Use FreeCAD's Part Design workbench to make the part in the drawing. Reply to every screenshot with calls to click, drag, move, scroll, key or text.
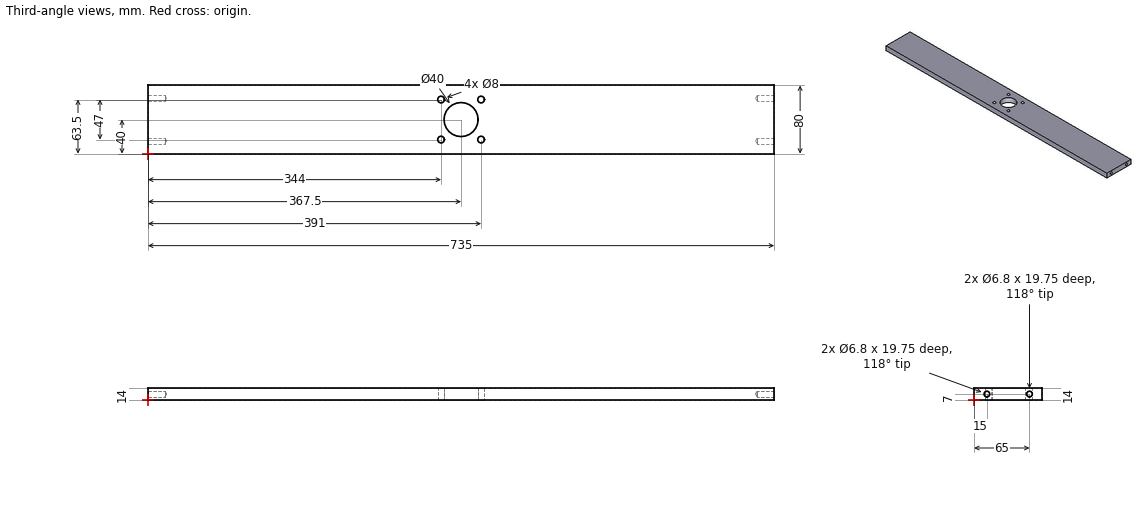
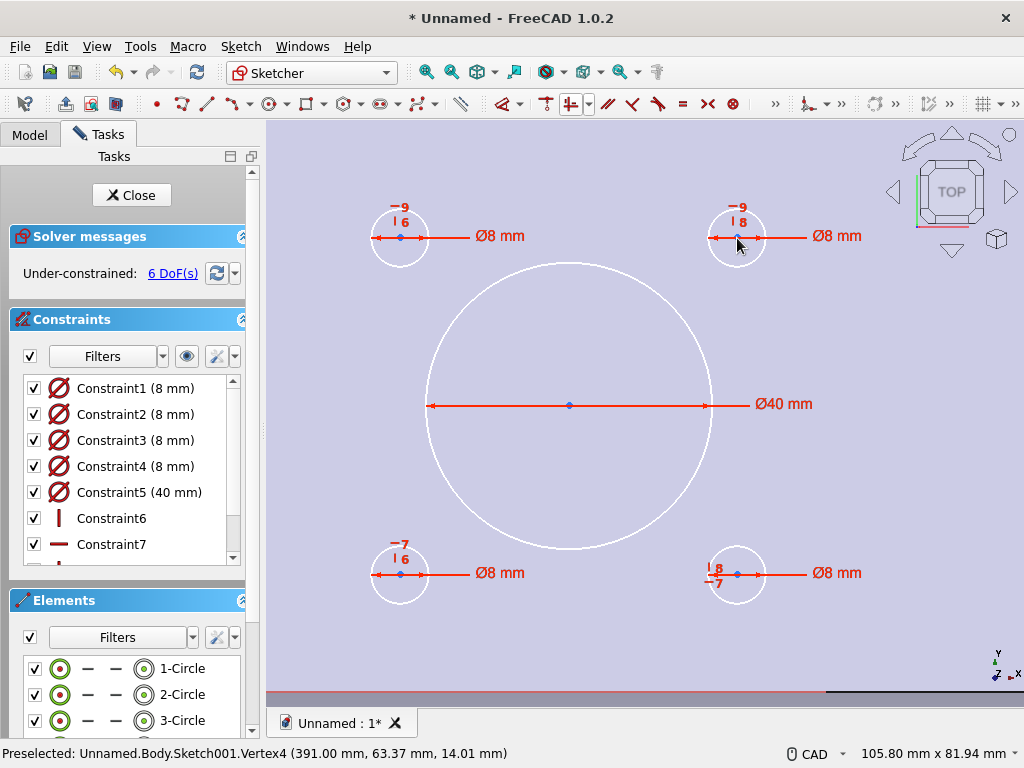
click(502, 104)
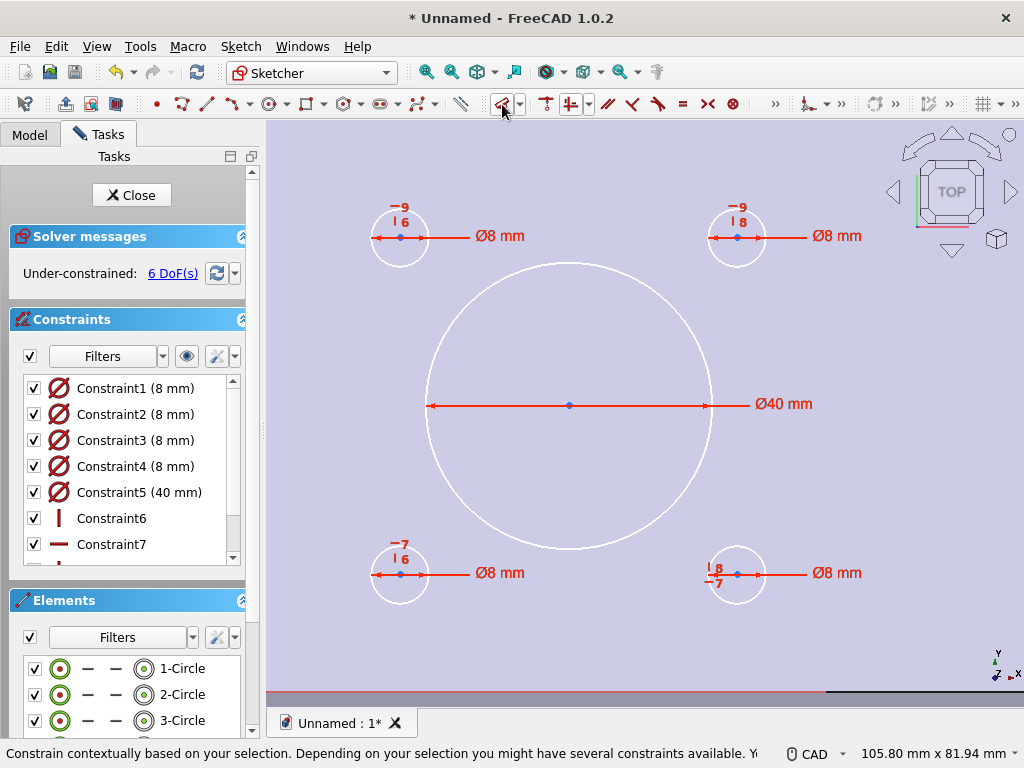
click(569, 406)
click(603, 480)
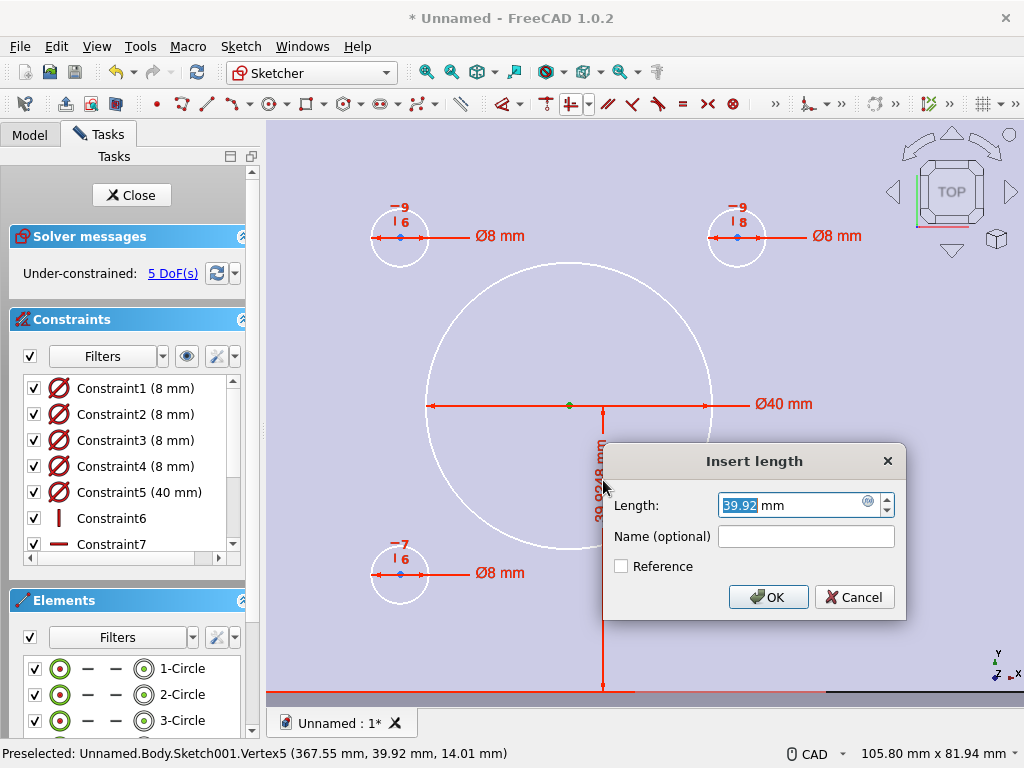
text(40)
key(Return)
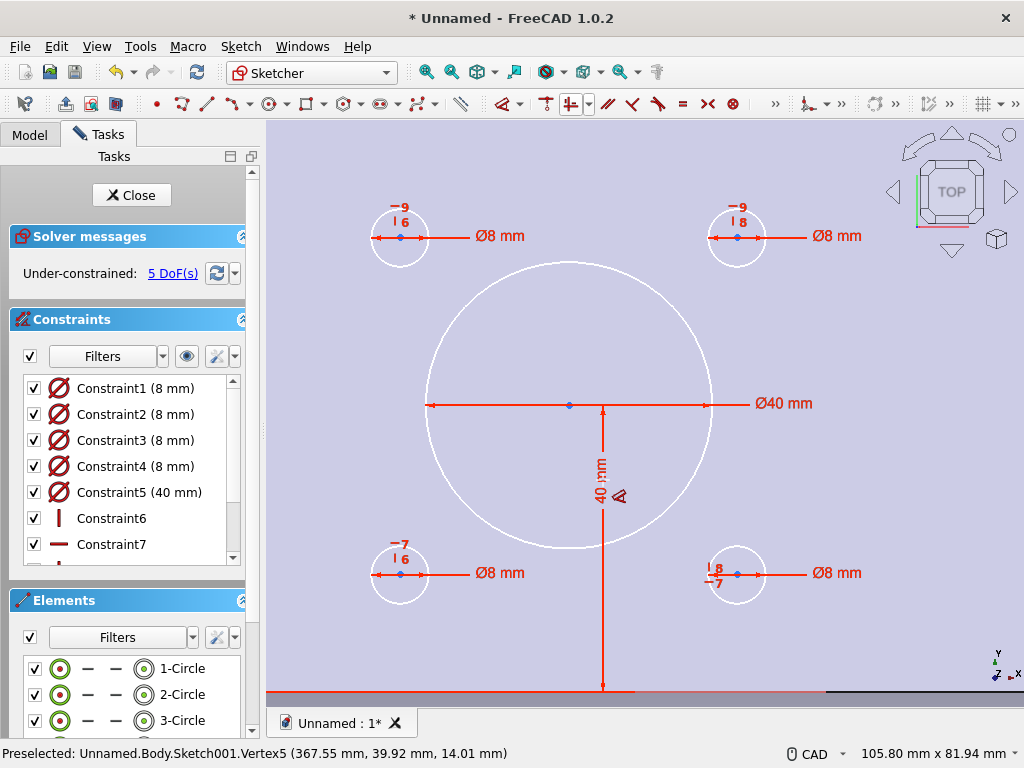
click(400, 238)
click(347, 204)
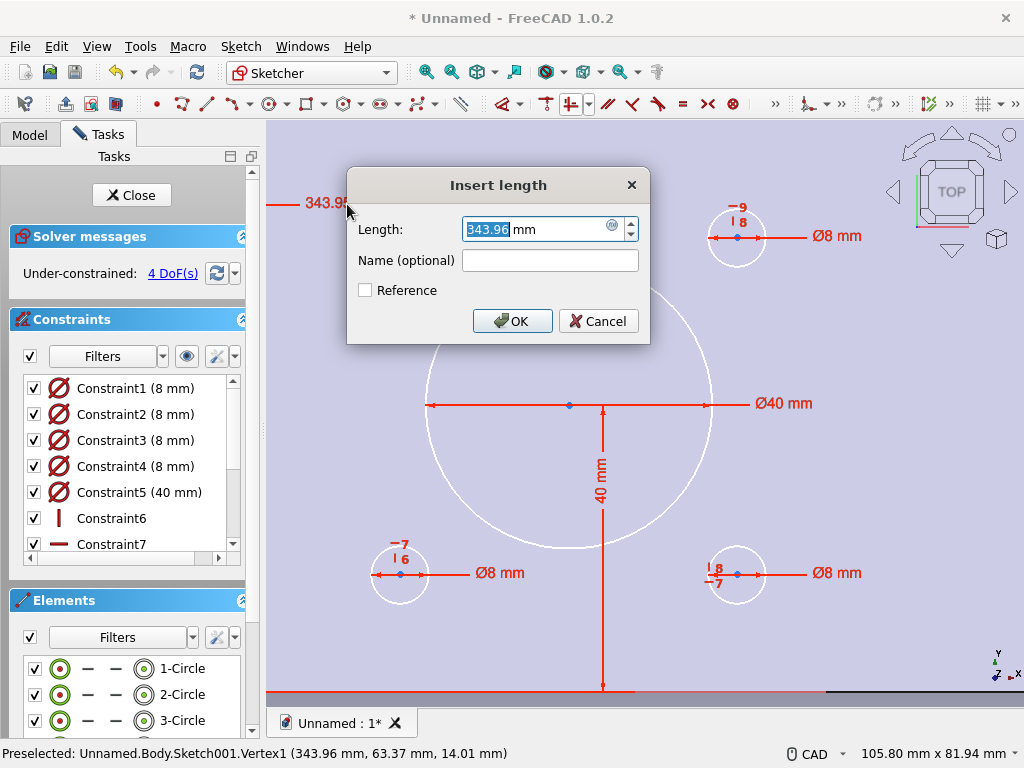
text(344)
key(Return)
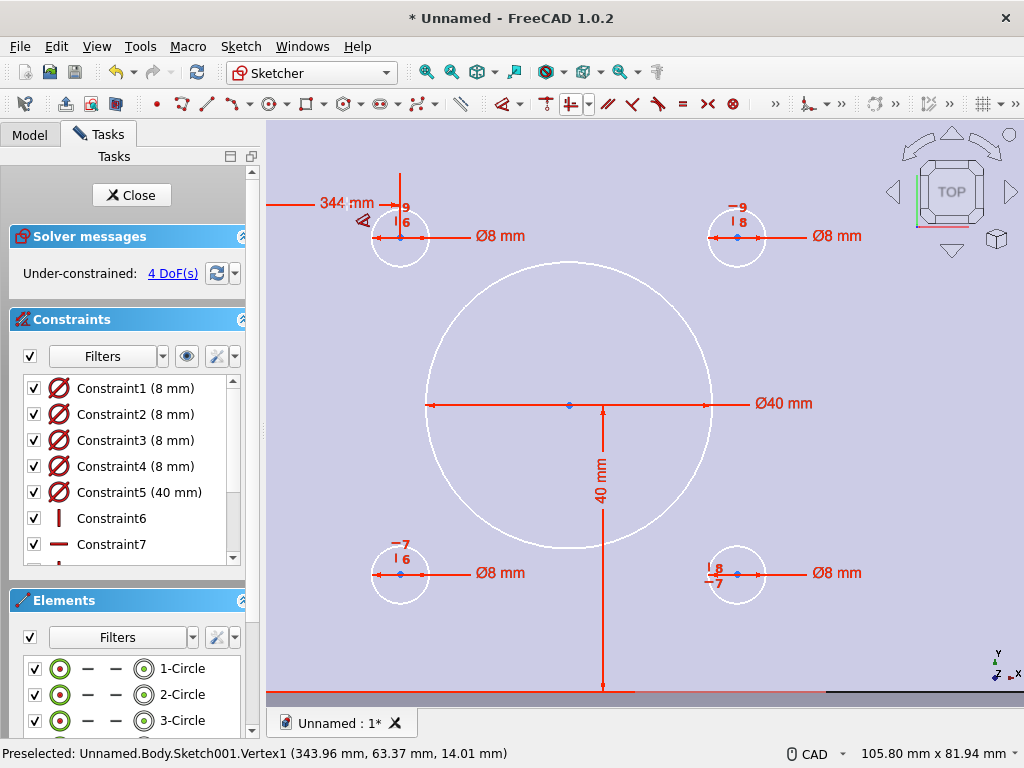
click(737, 575)
click(360, 541)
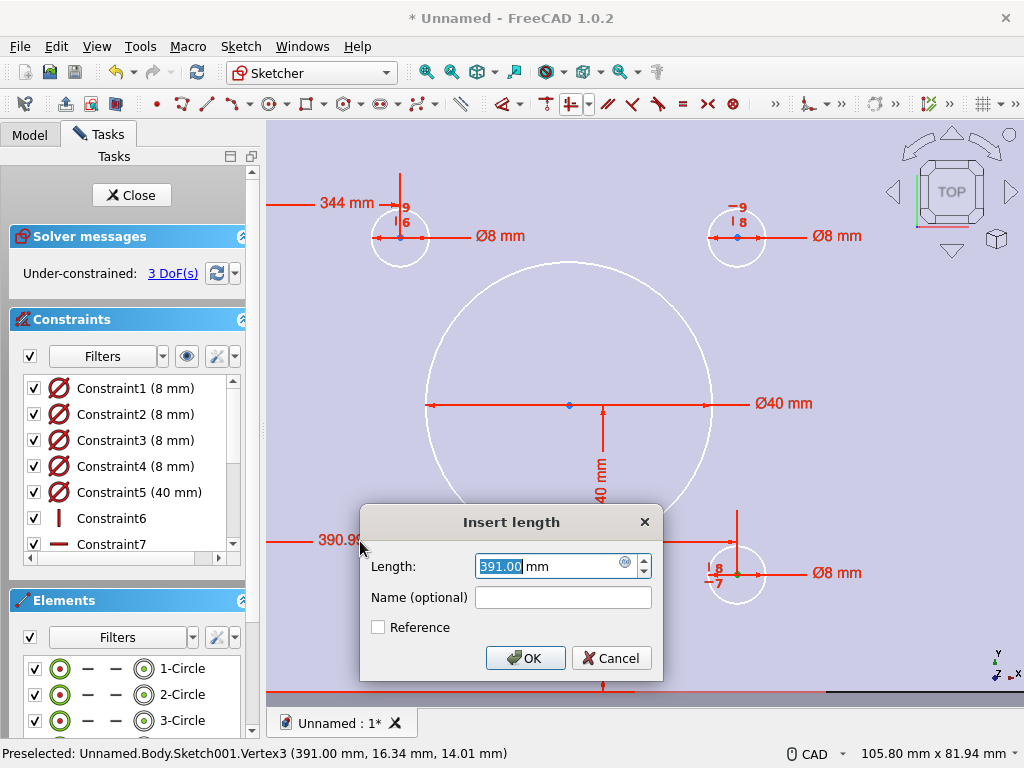
text(391)
key(Return)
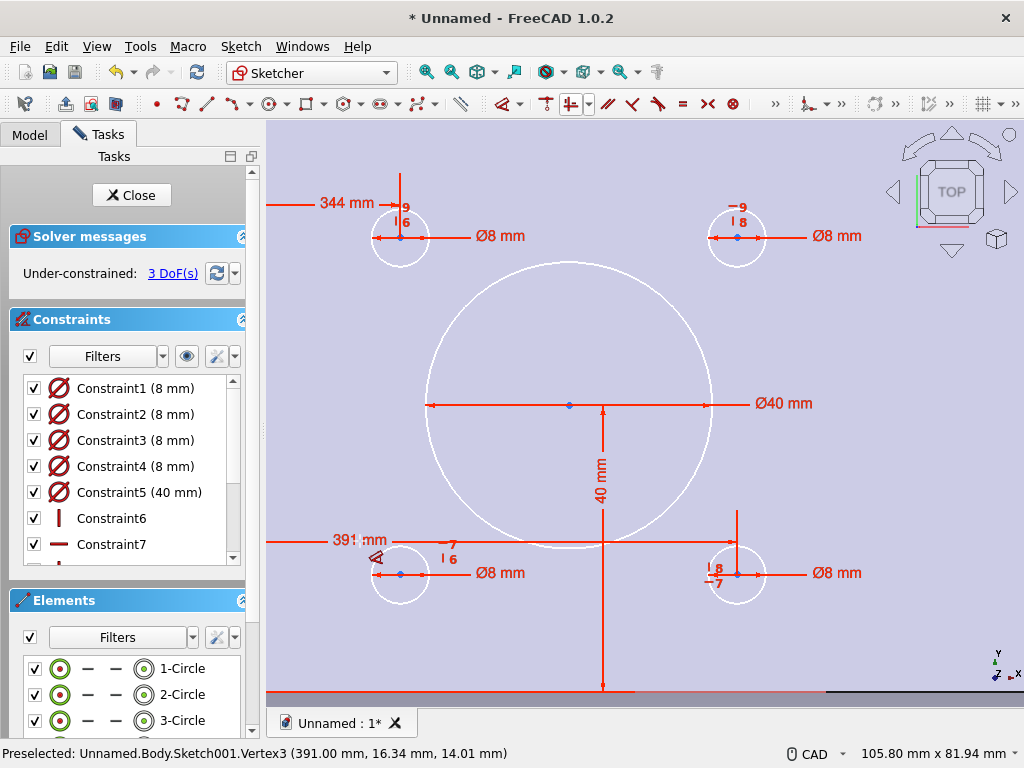
click(400, 238)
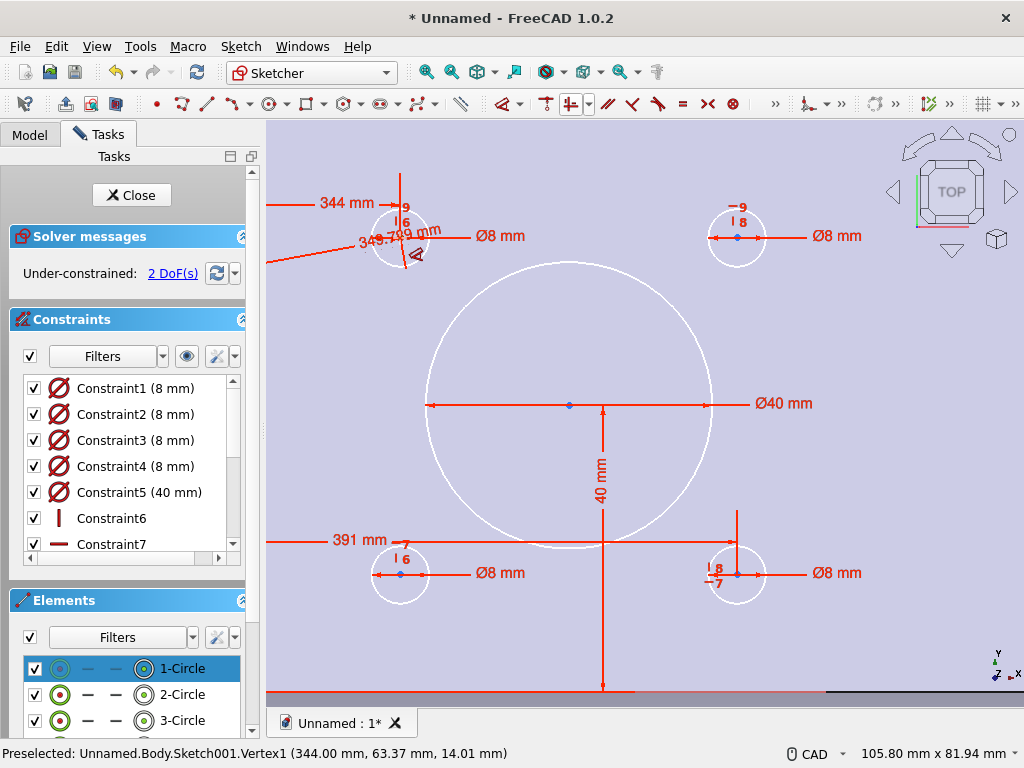
click(400, 575)
click(366, 406)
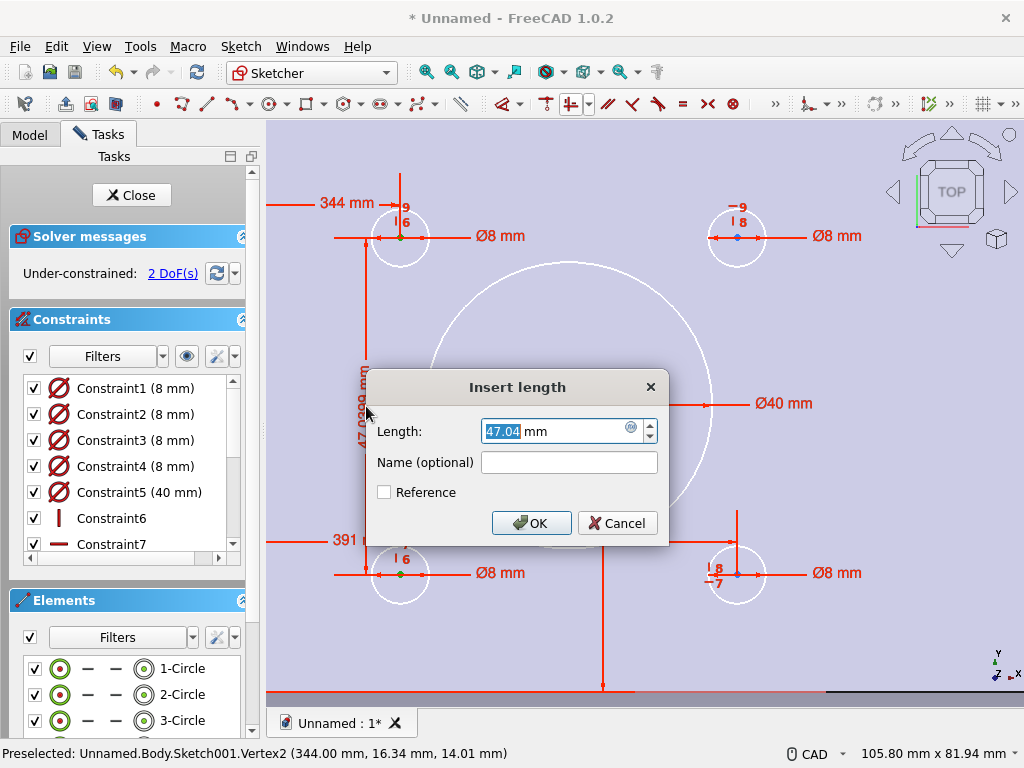
text(47)
key(Return)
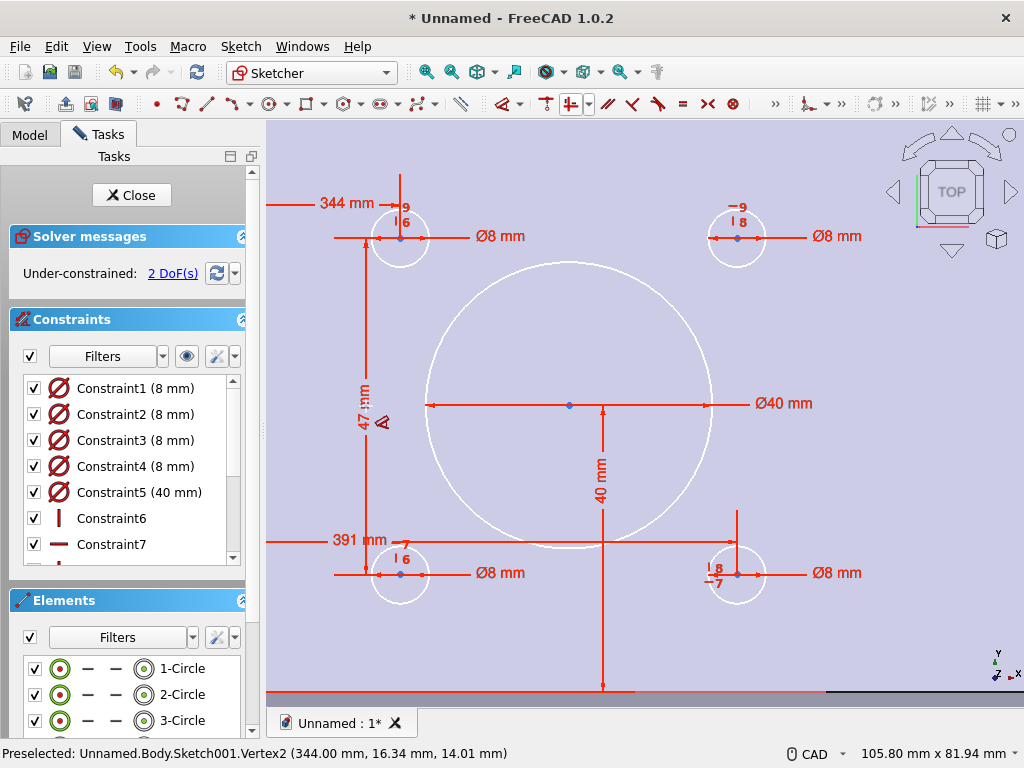
click(400, 238)
click(434, 304)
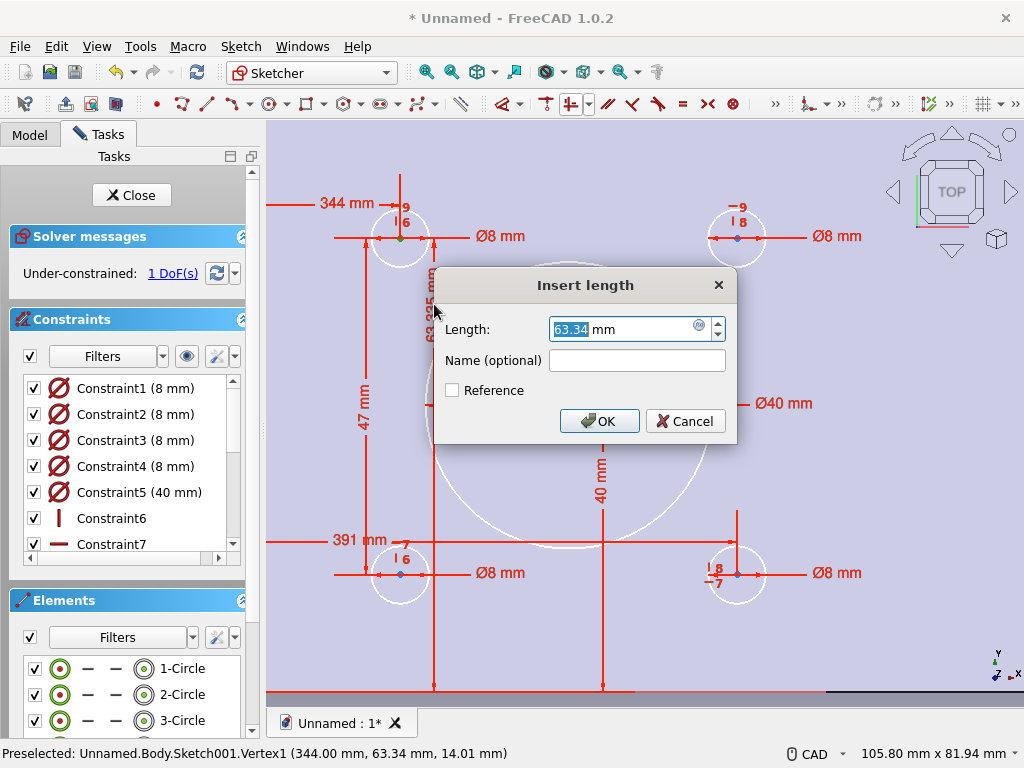
text(63.5)
key(Return)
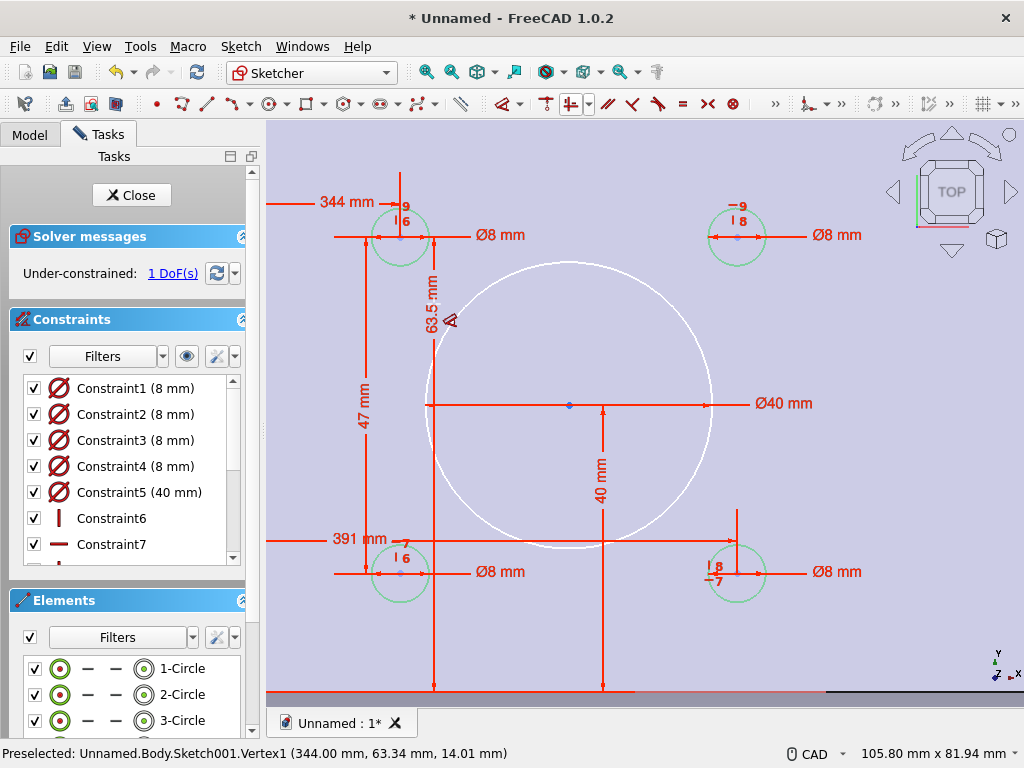
click(569, 405)
click(368, 371)